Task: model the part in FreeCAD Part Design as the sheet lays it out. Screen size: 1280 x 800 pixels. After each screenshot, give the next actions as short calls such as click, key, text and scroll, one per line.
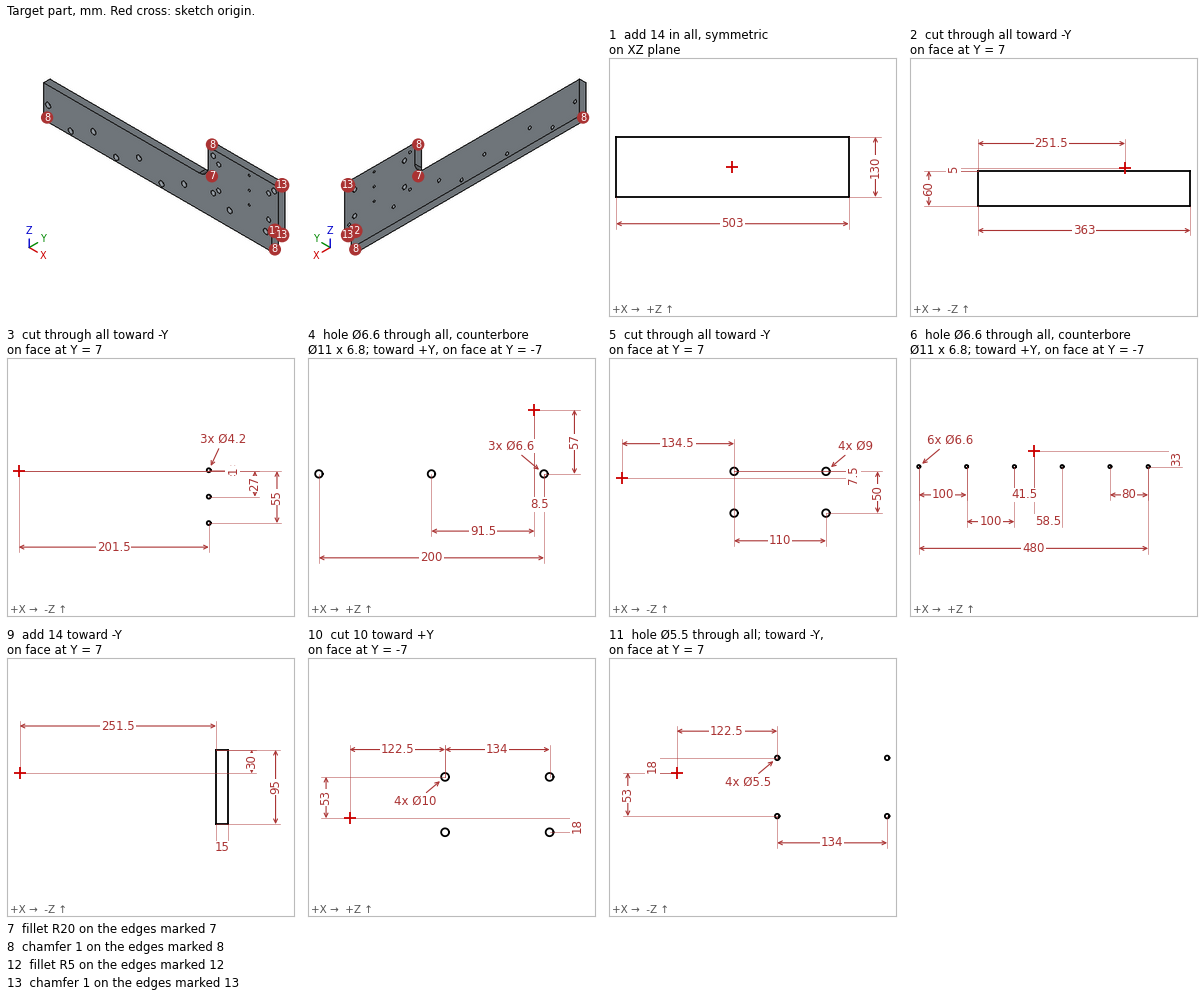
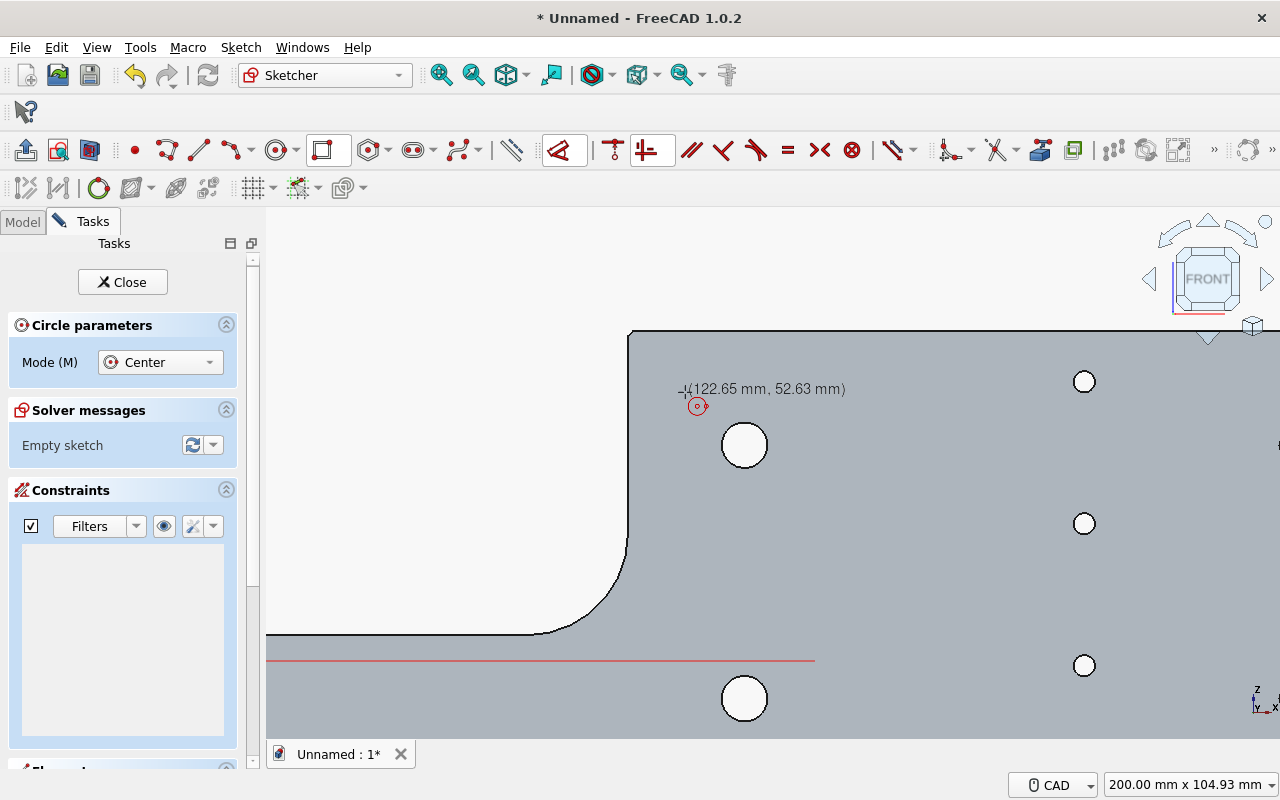
click(684, 392)
click(702, 374)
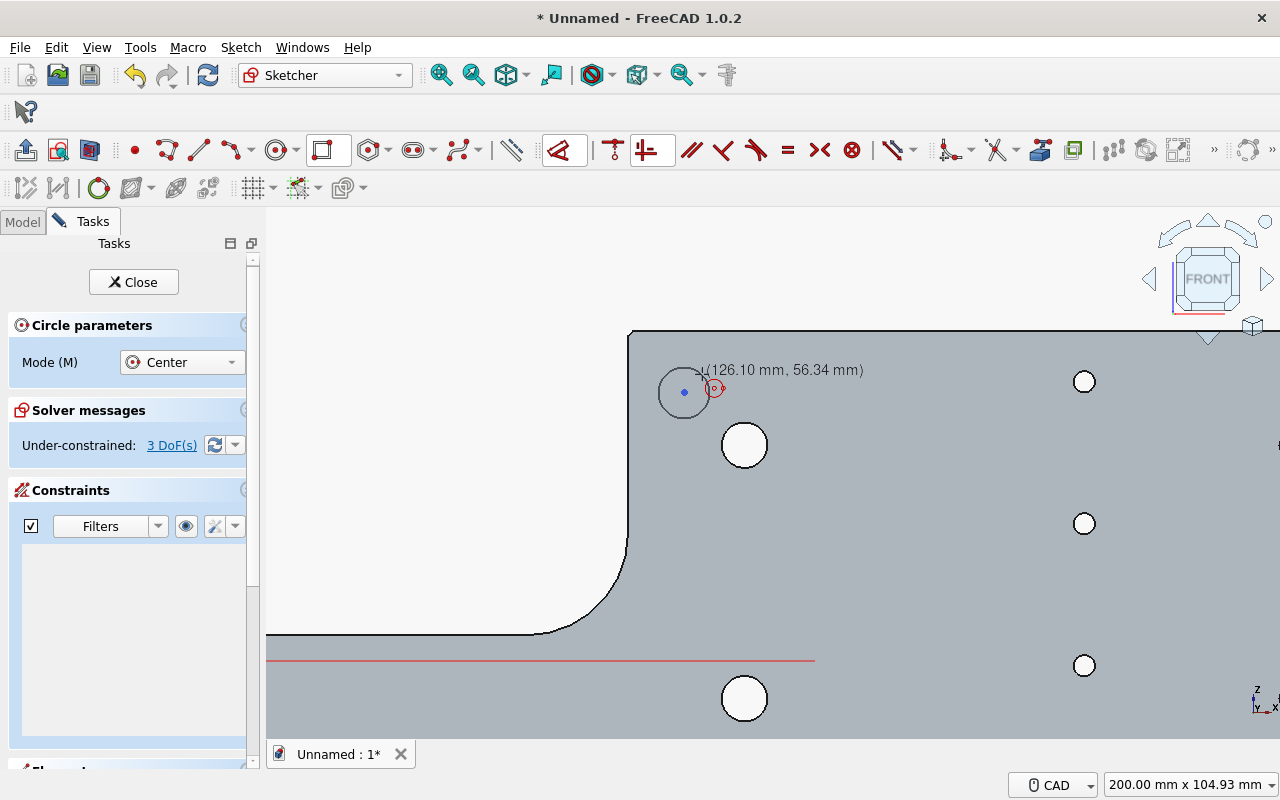
scroll(687, 392, down, 4)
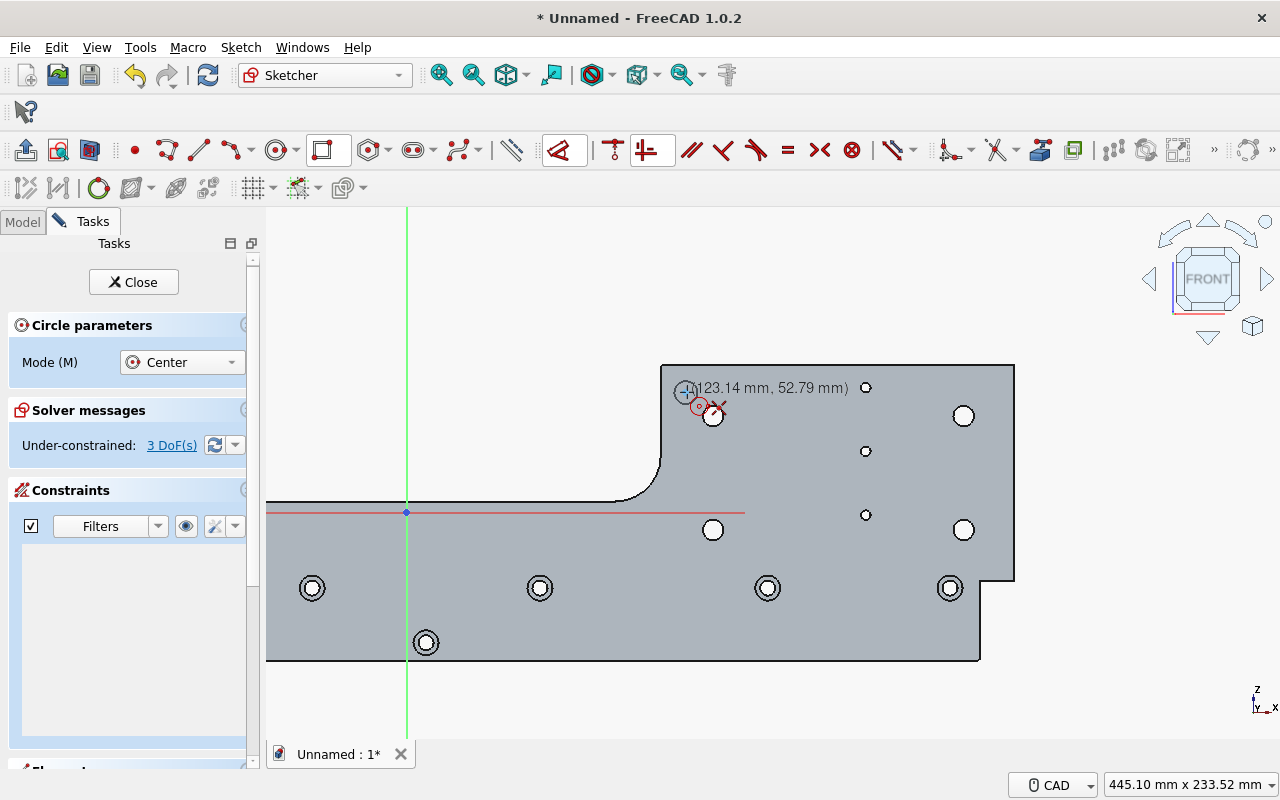
scroll(991, 392, up, 4)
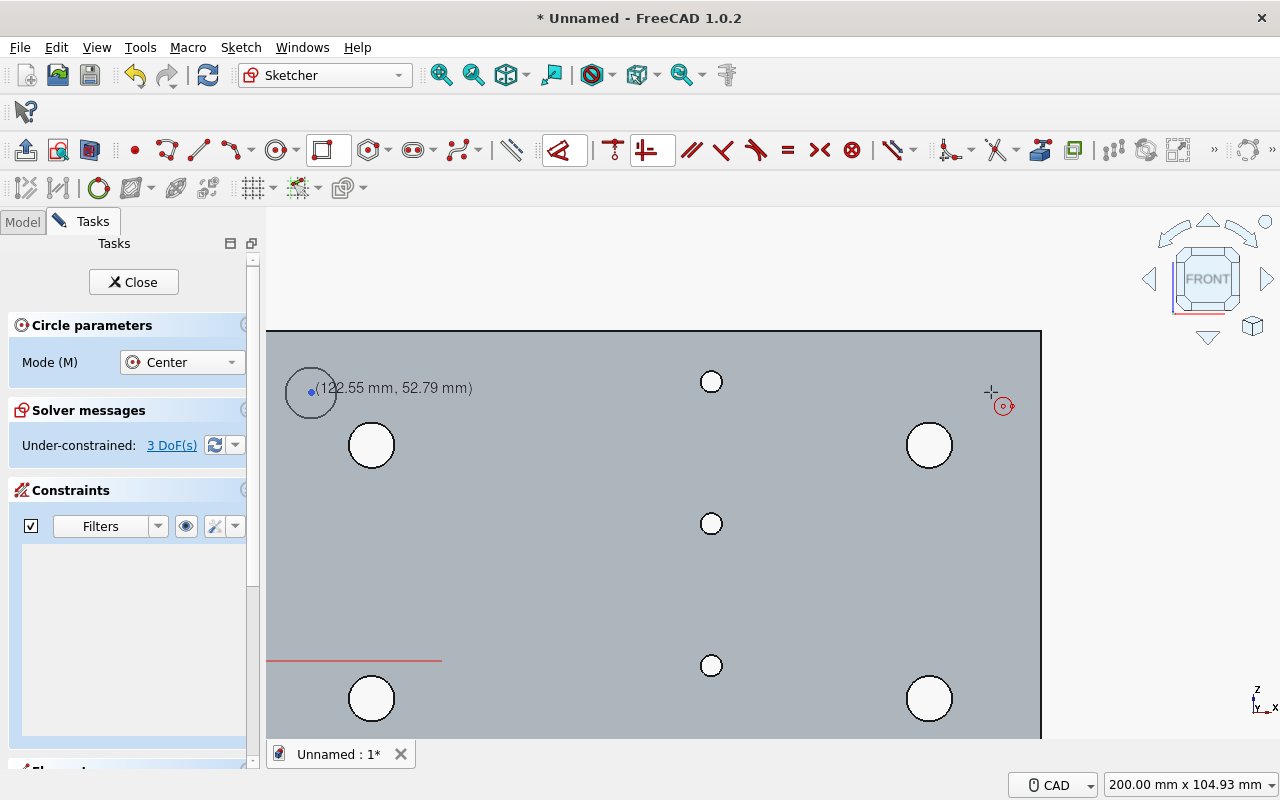
click(990, 392)
click(1008, 374)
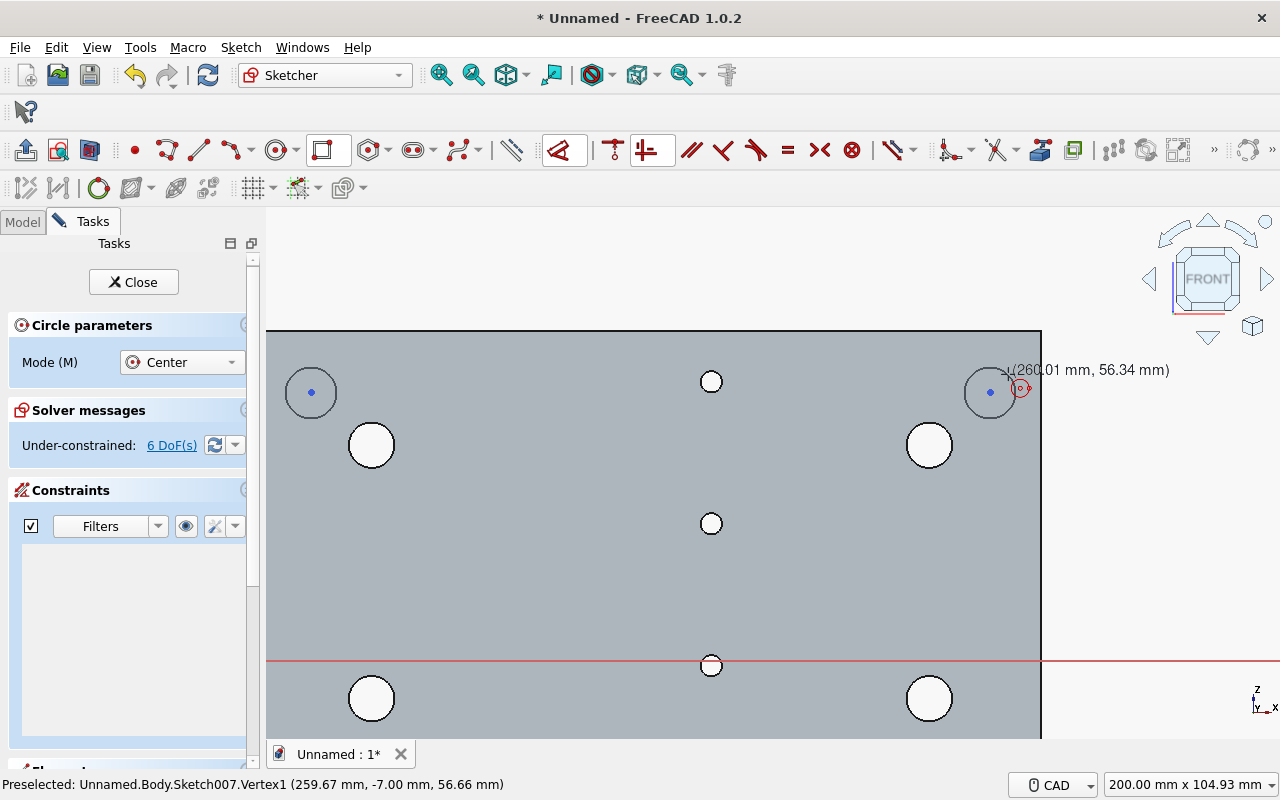
scroll(992, 392, down, 4)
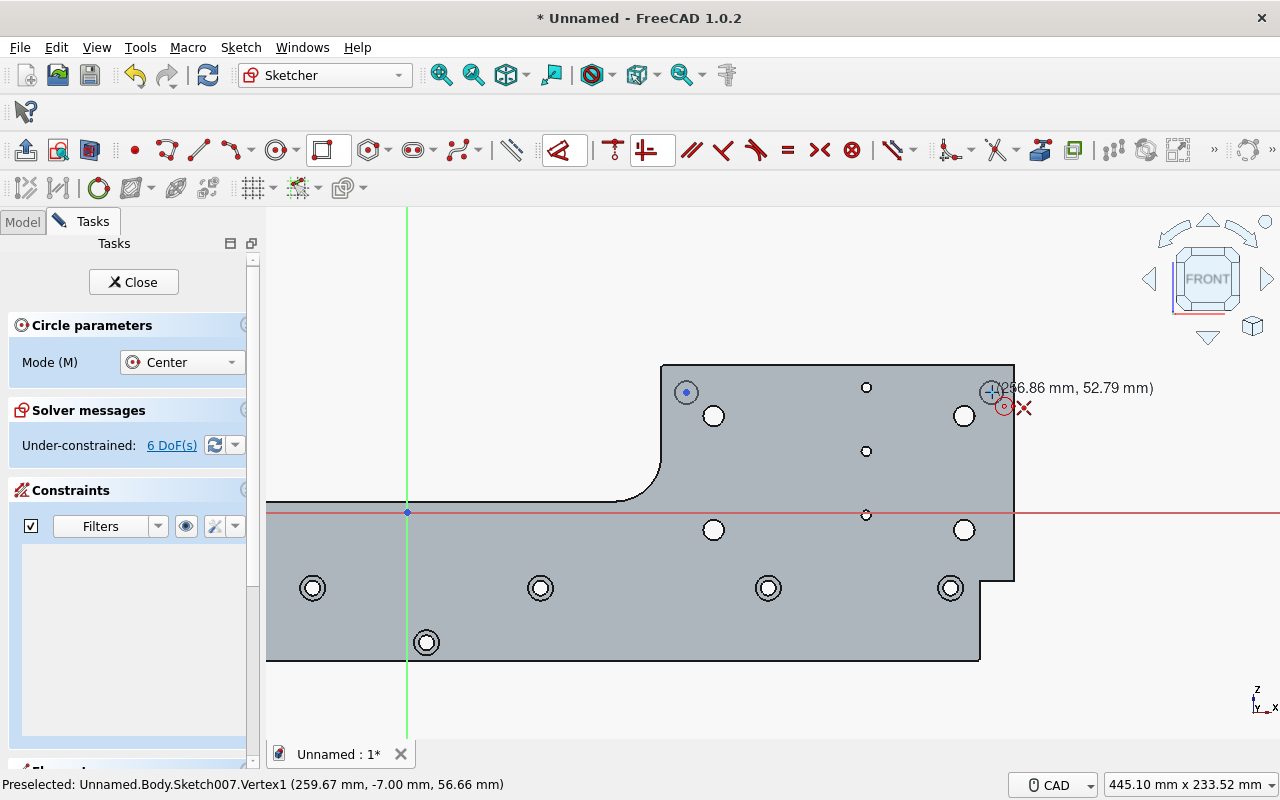
scroll(992, 554, up, 4)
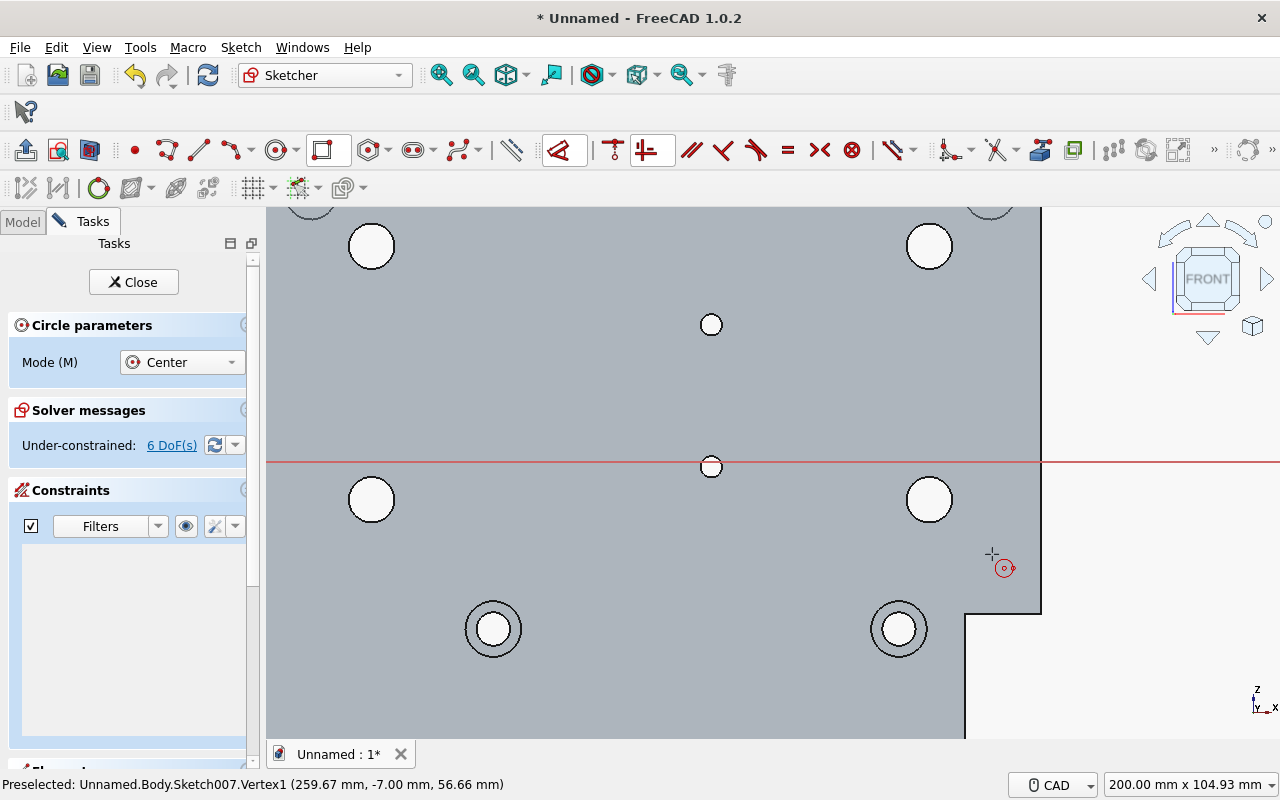
click(990, 553)
click(1008, 535)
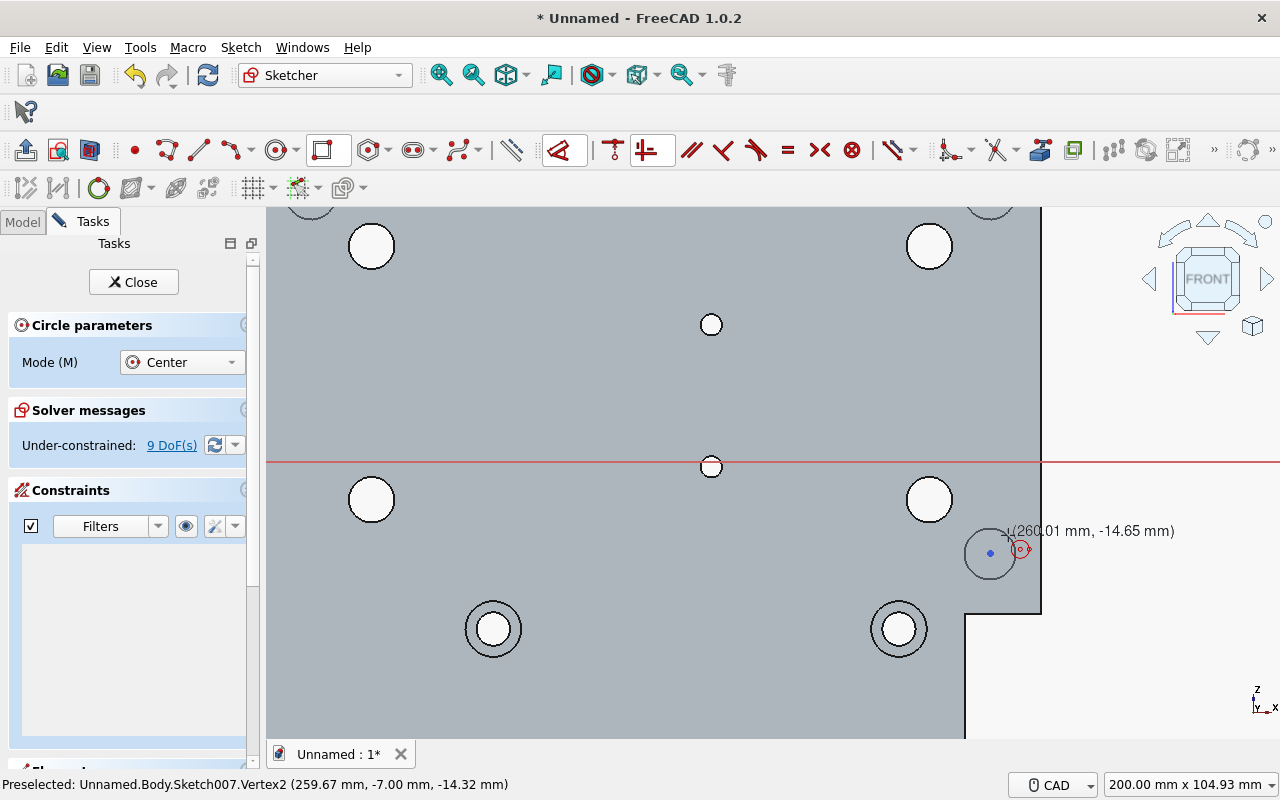
click(311, 553)
click(329, 535)
key(Escape)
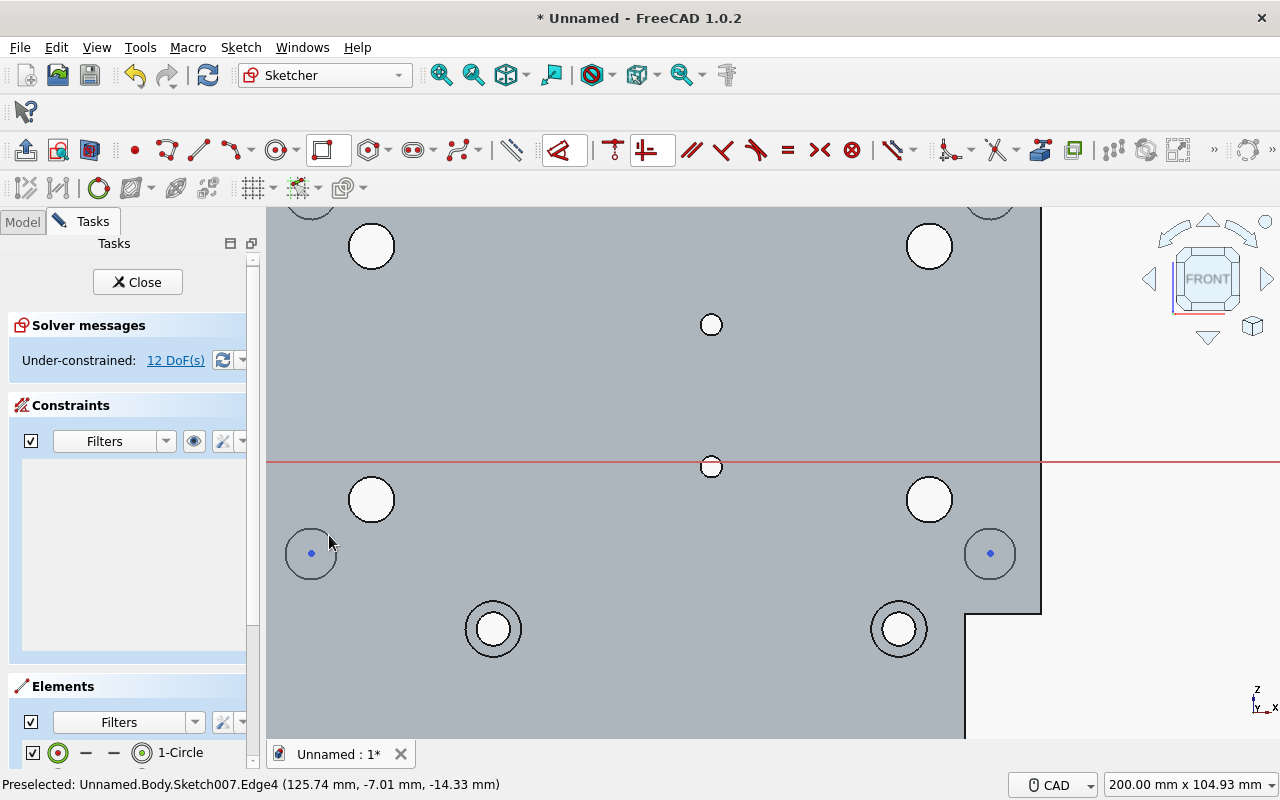
scroll(992, 555, down, 4)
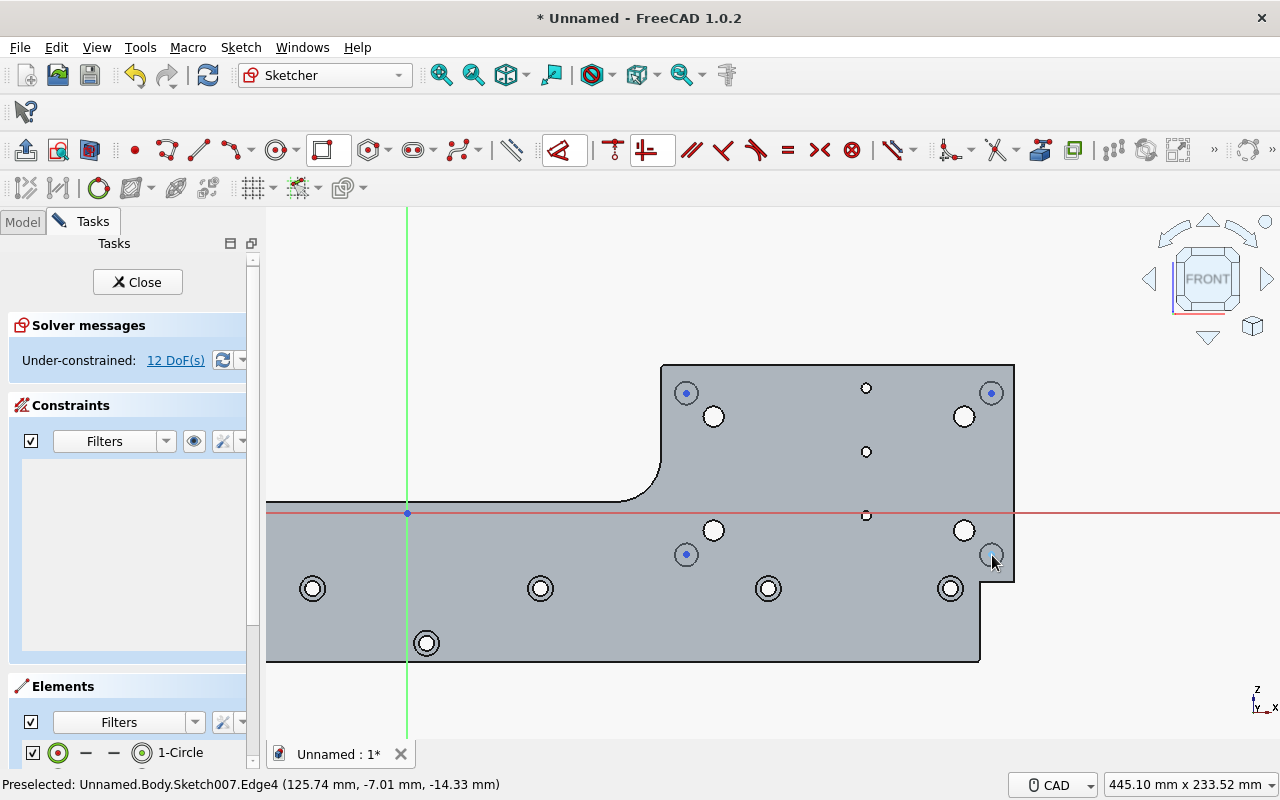
click(694, 385)